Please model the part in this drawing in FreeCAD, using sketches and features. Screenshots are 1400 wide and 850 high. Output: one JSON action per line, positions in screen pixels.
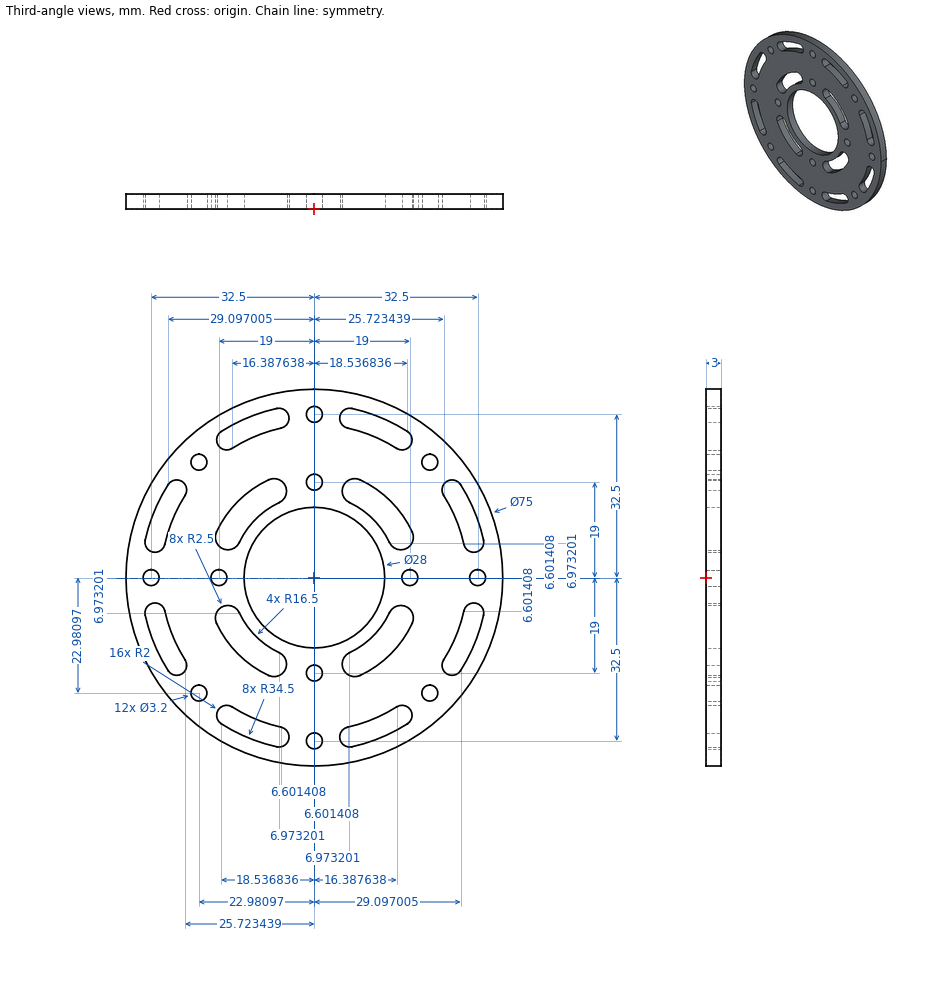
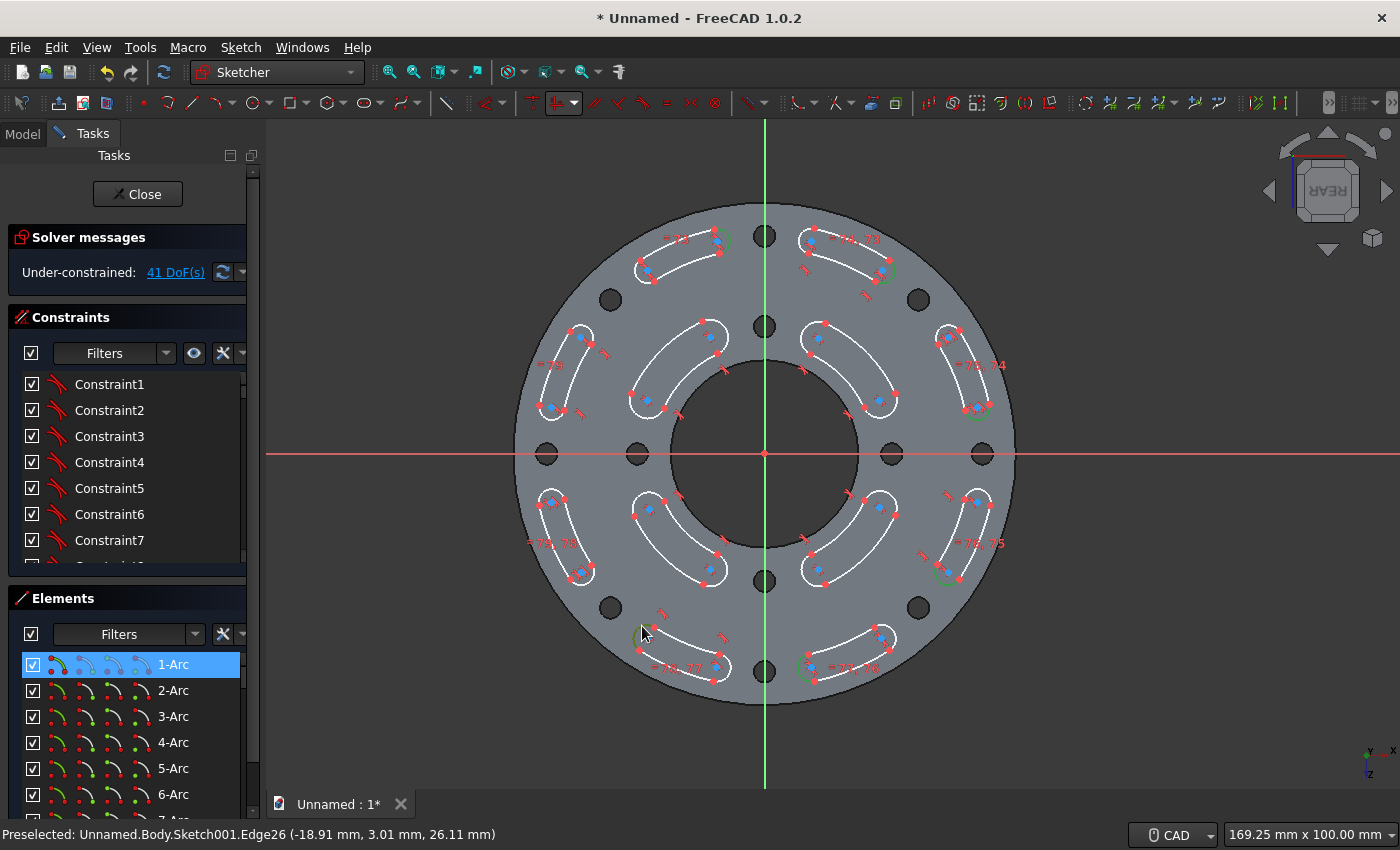
{"action": "left_click", "coordinate": [557, 490]}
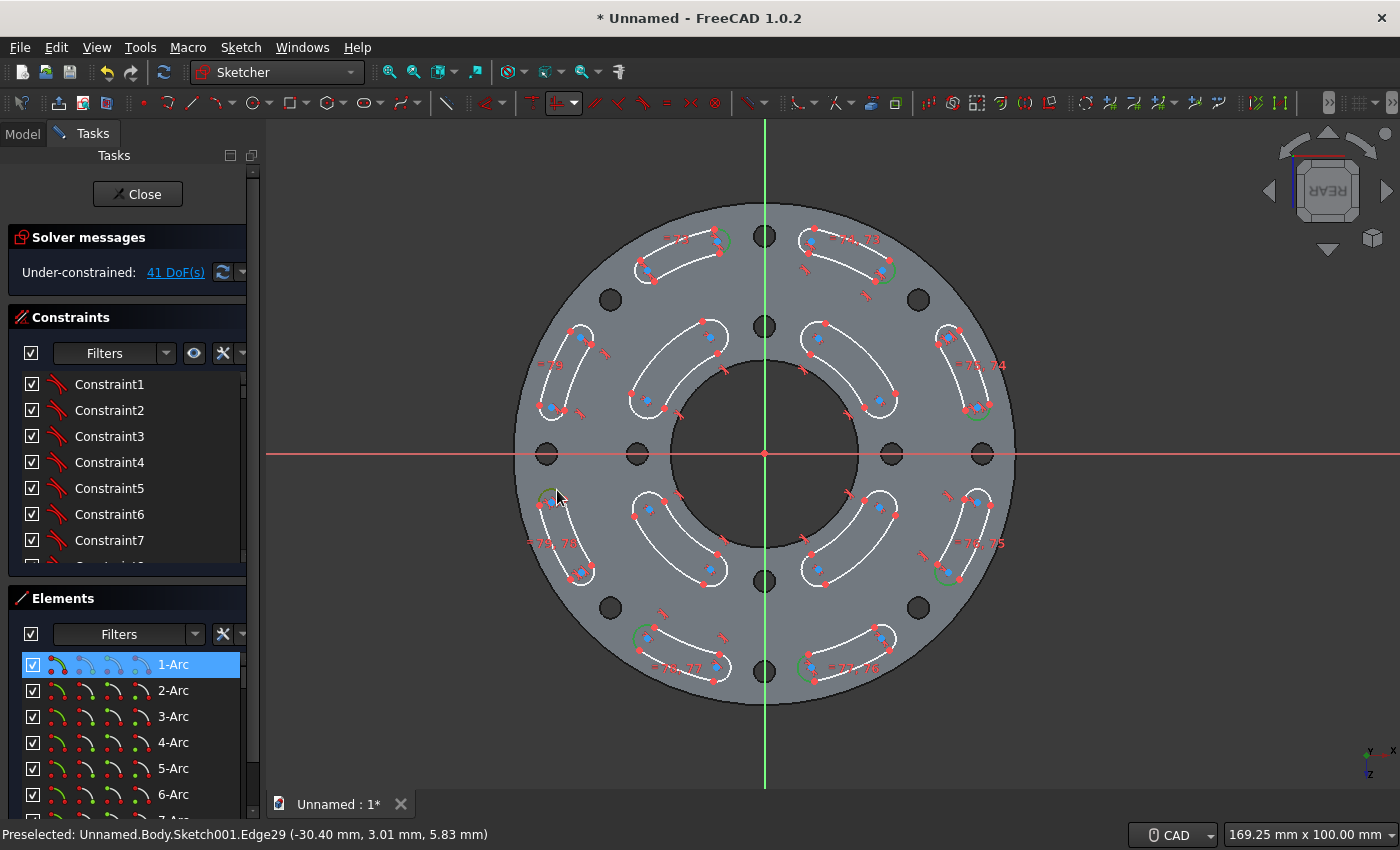
{"action": "scroll", "coordinate": [592, 333], "scroll_direction": "up", "scroll_amount": 2}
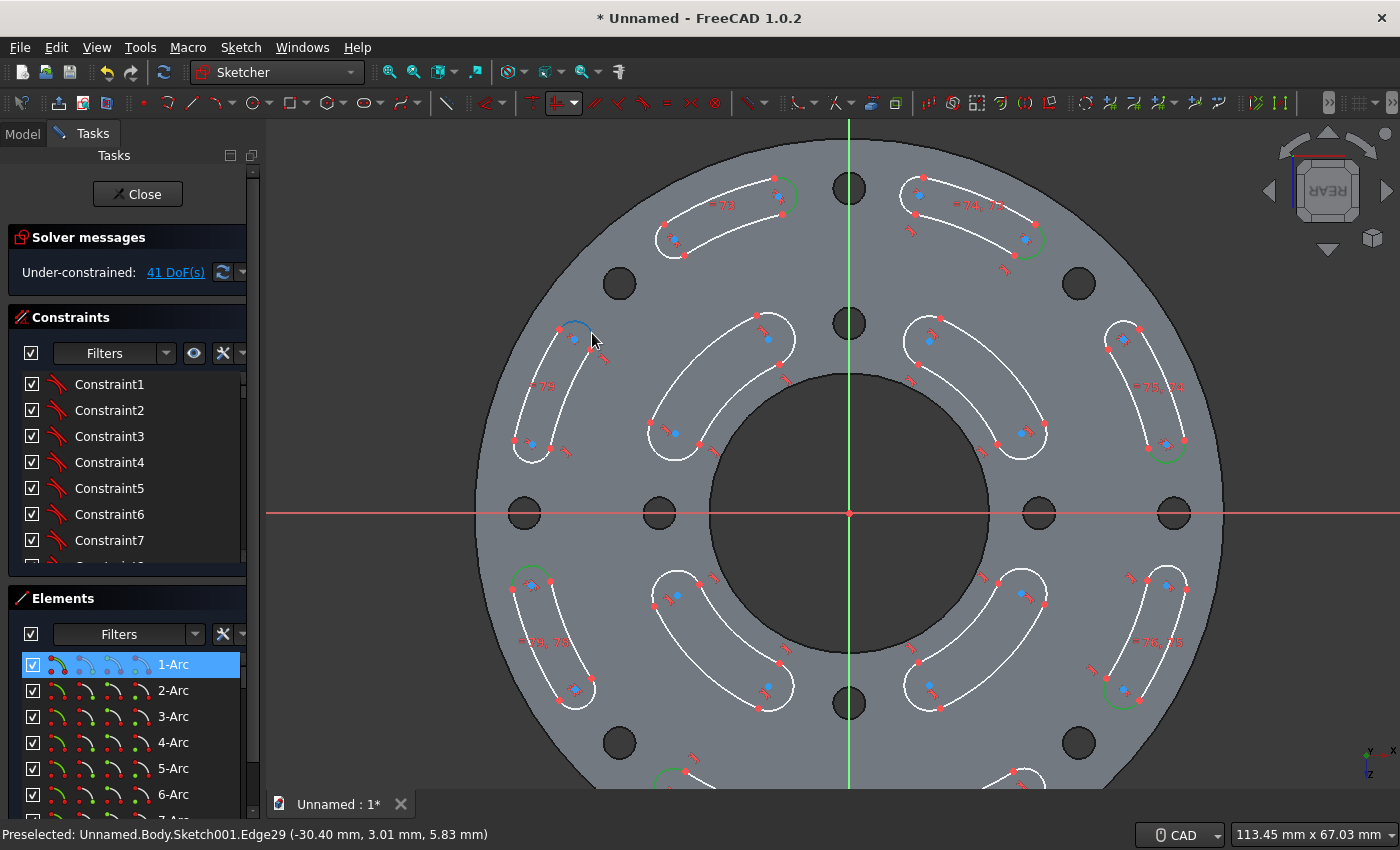
{"action": "left_click", "coordinate": [592, 333]}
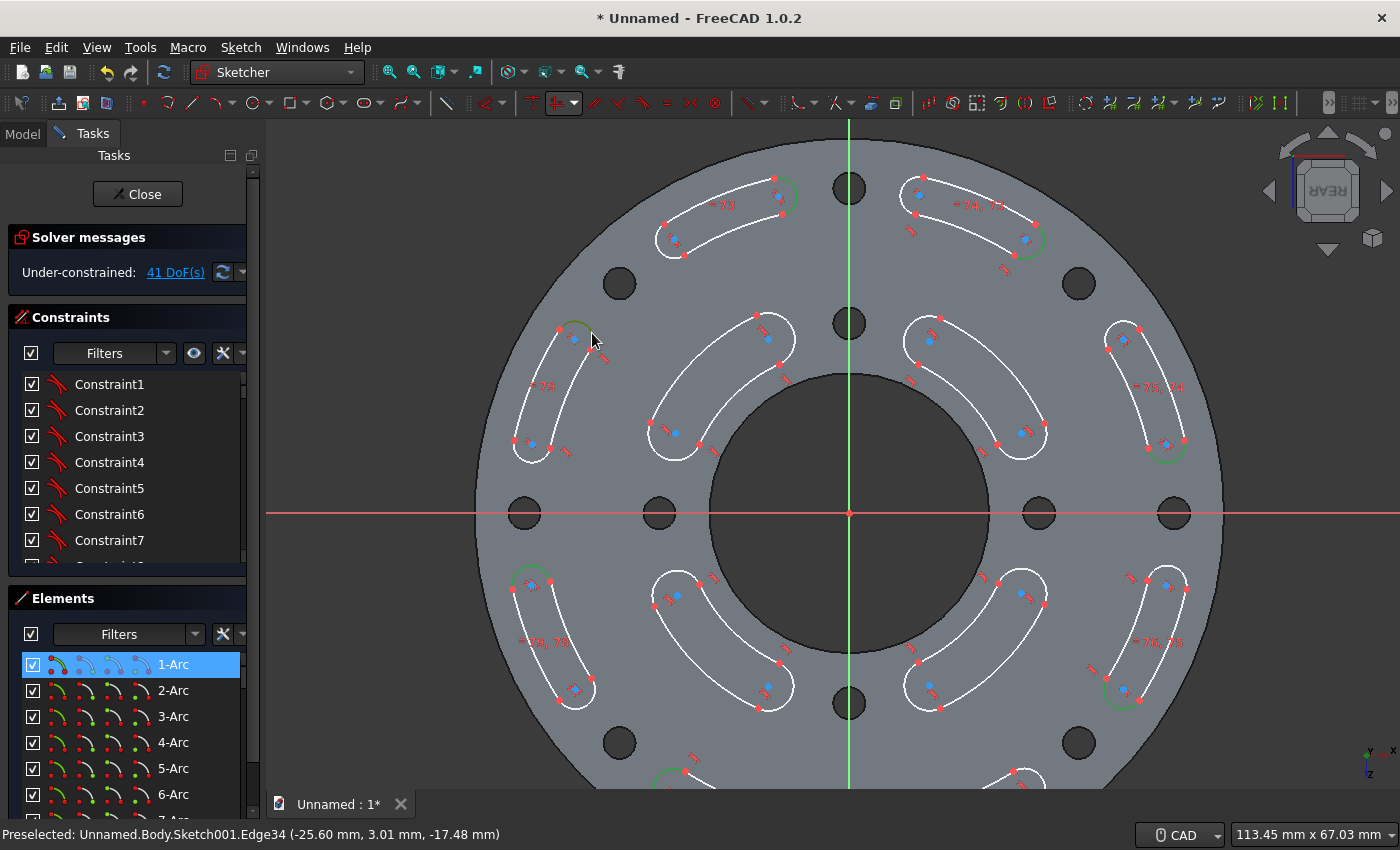
{"action": "left_click", "coordinate": [668, 104]}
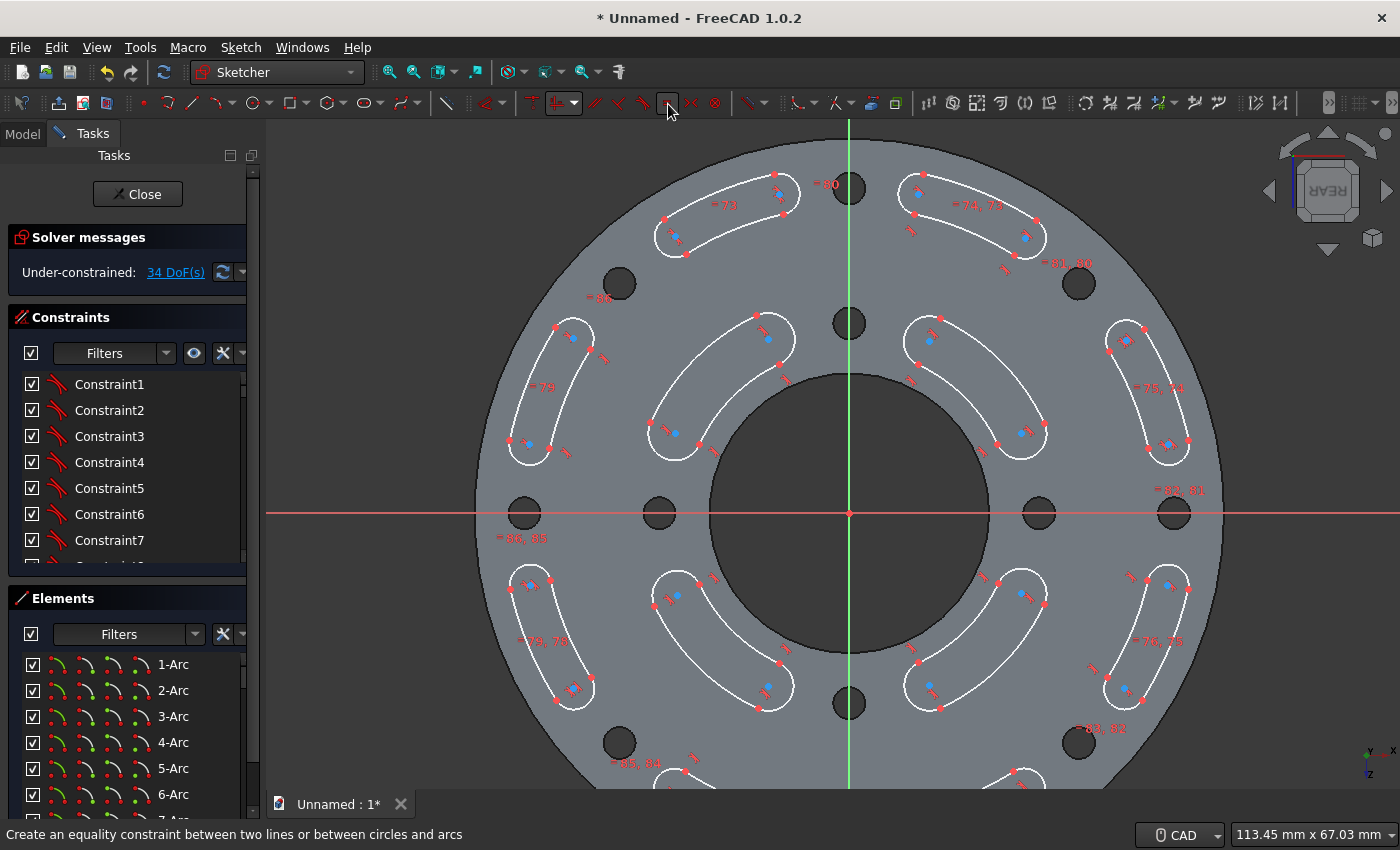
{"action": "left_click", "coordinate": [750, 382]}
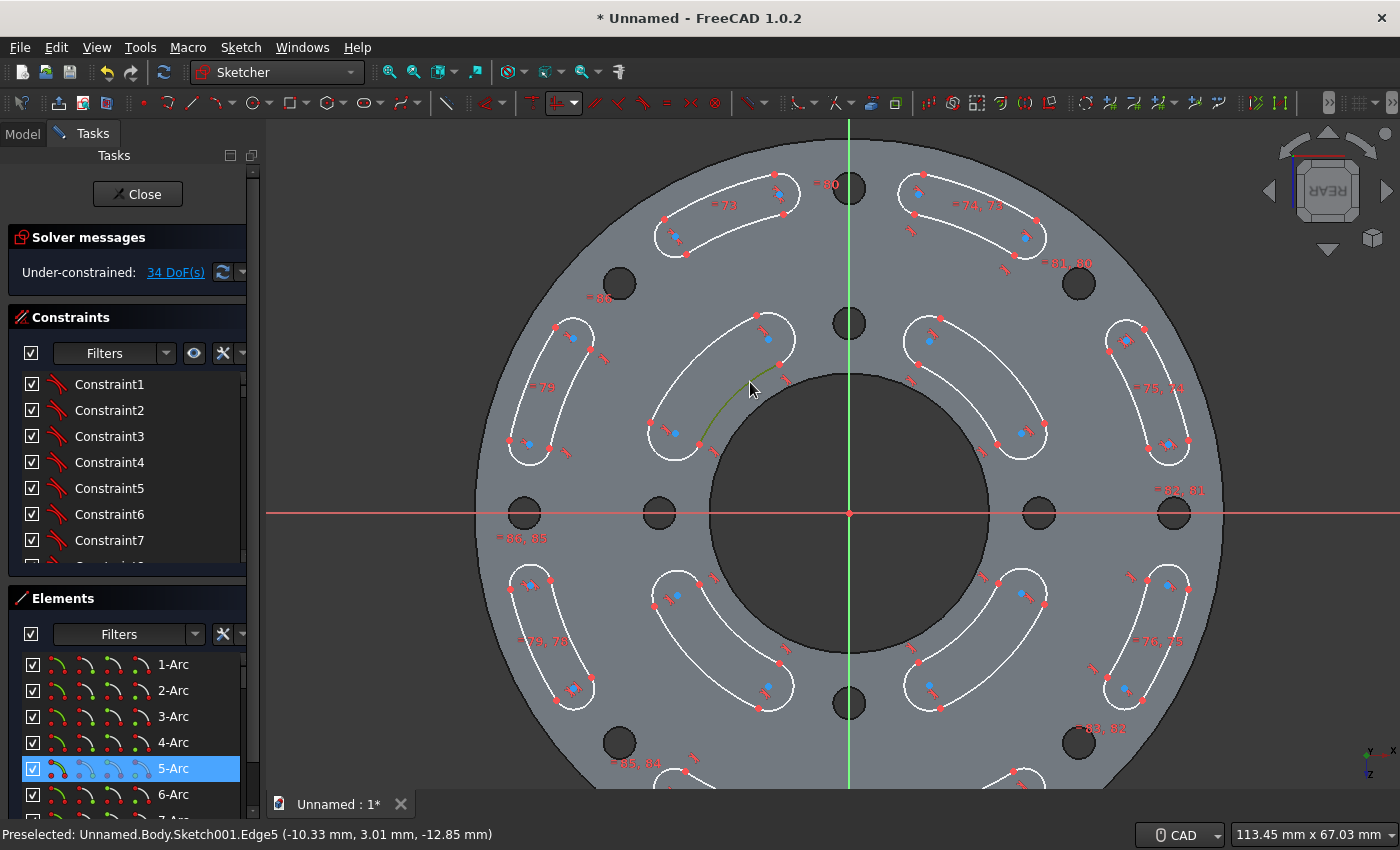
{"action": "left_click", "coordinate": [980, 415]}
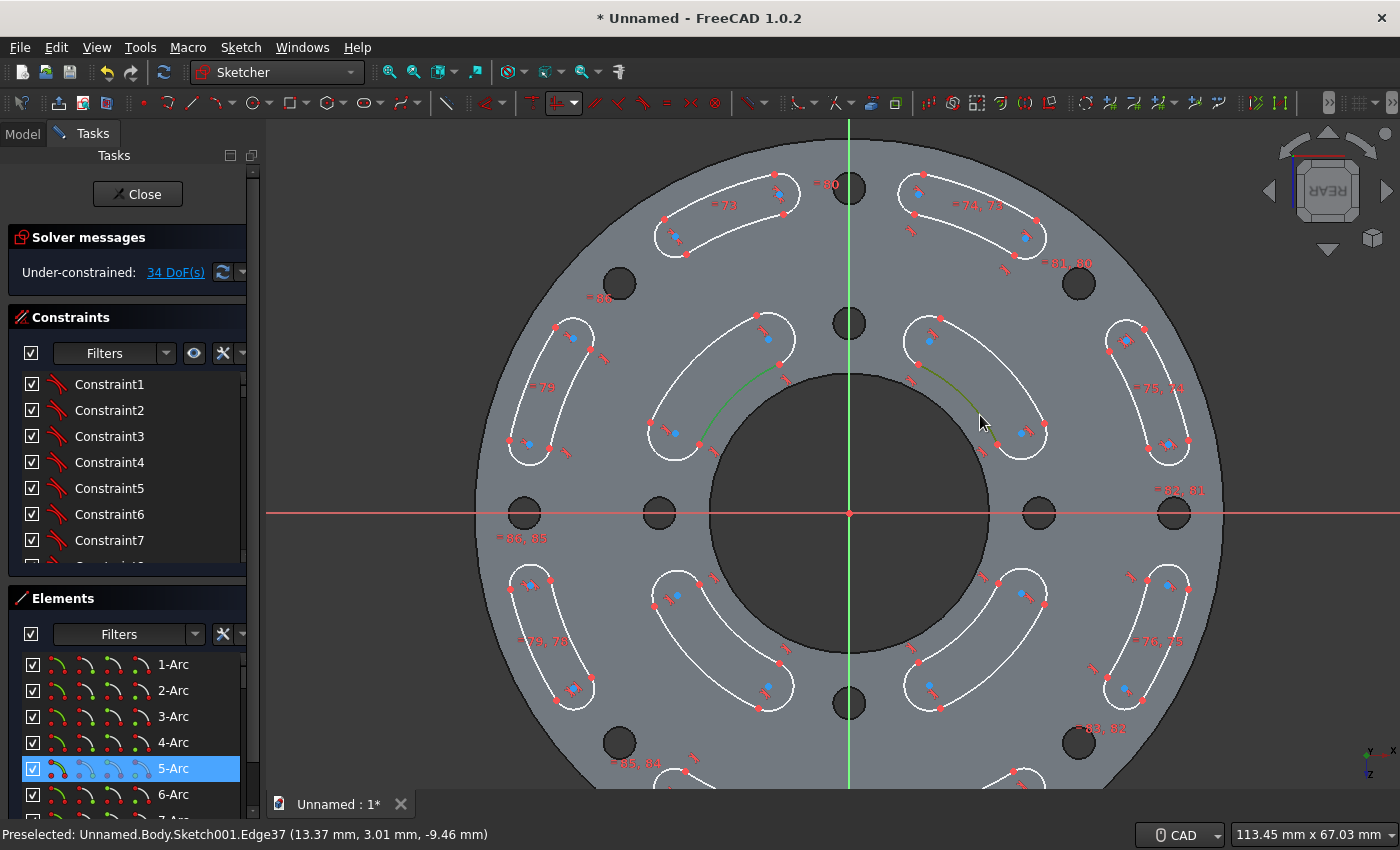
{"action": "left_click", "coordinate": [948, 645]}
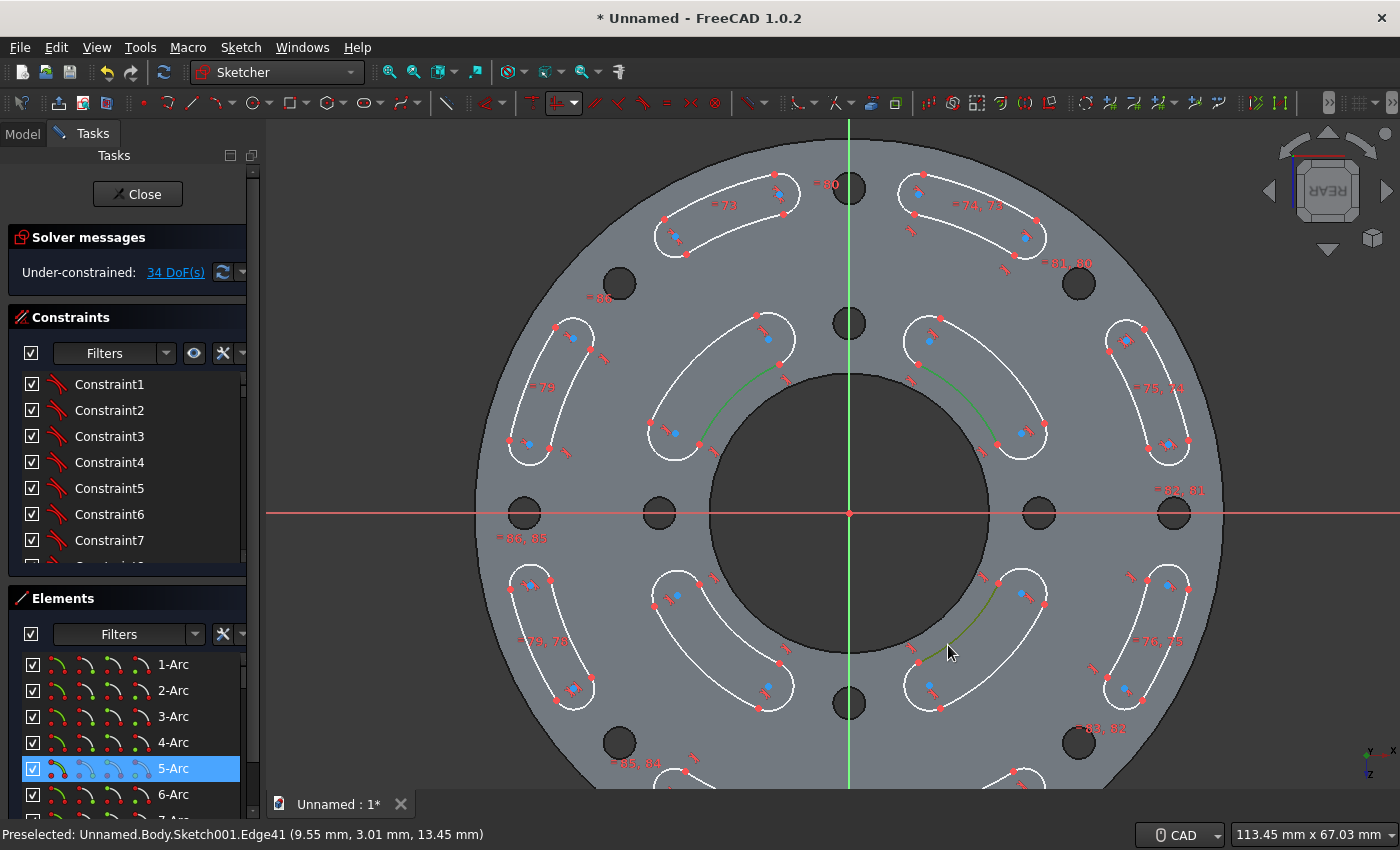
{"action": "left_click", "coordinate": [718, 614]}